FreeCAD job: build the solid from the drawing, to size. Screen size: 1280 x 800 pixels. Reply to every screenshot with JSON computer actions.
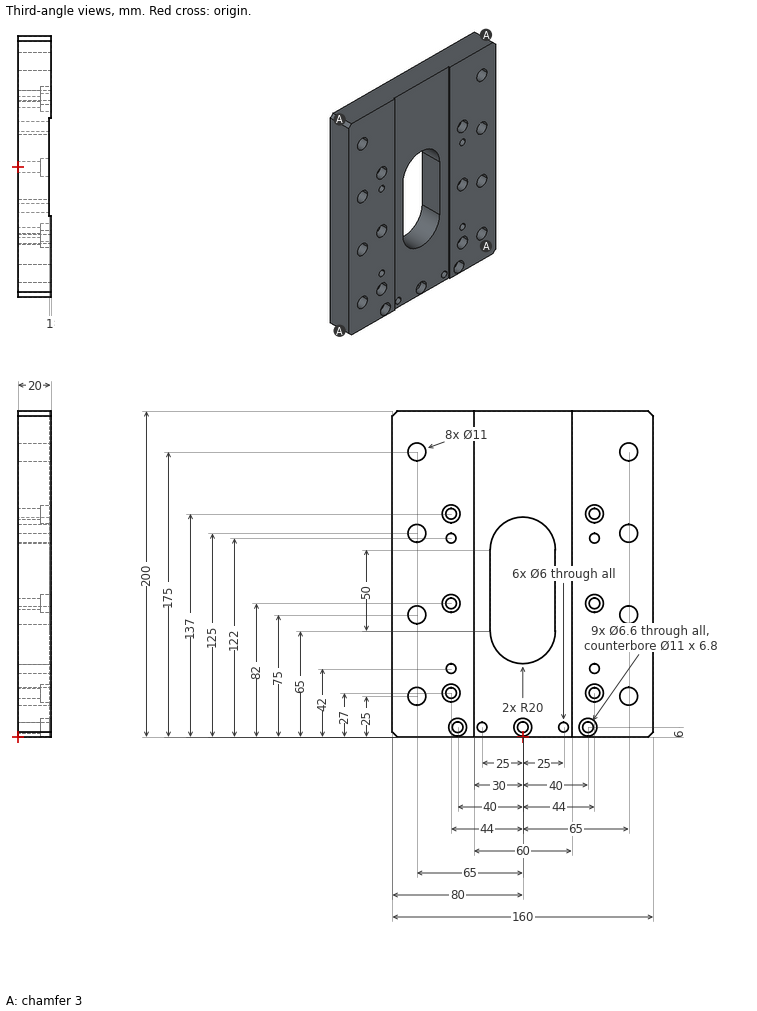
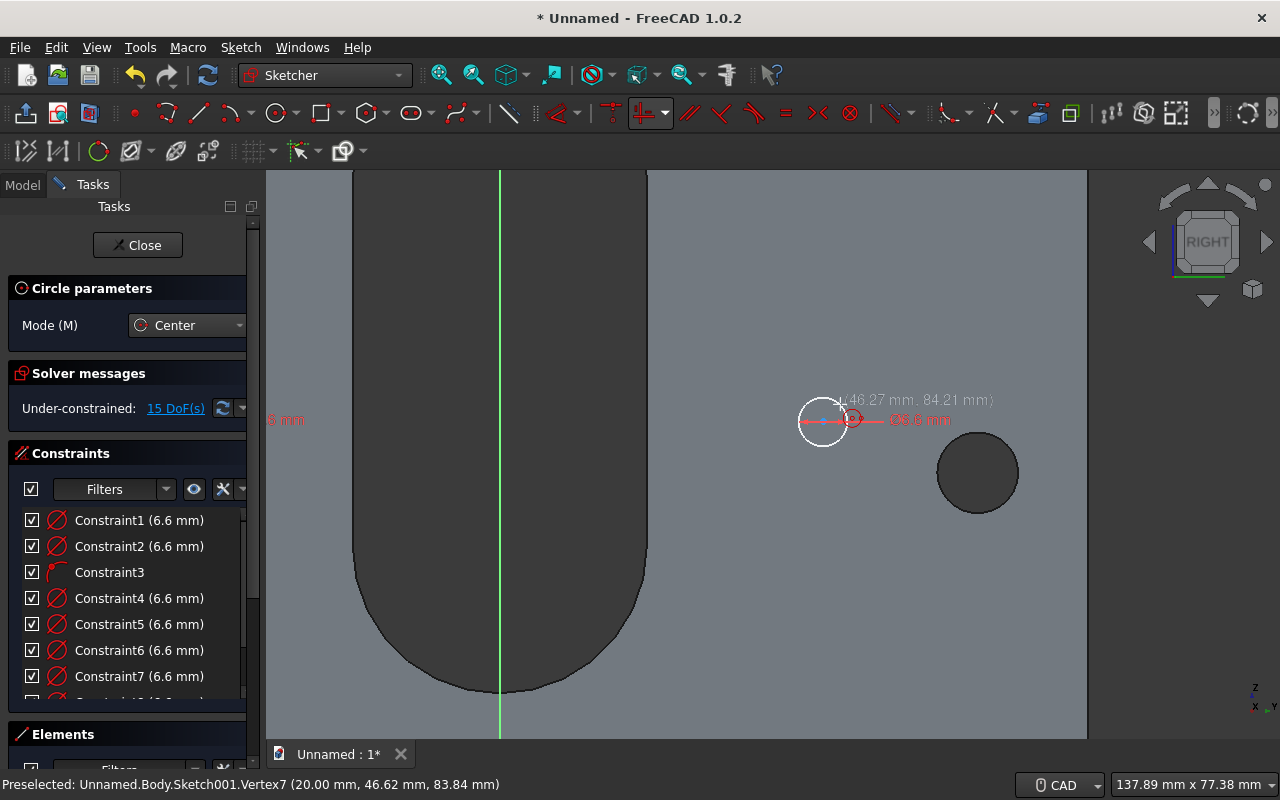
{"action": "scroll", "coordinate": [824, 423], "scroll_direction": "down", "scroll_amount": 5}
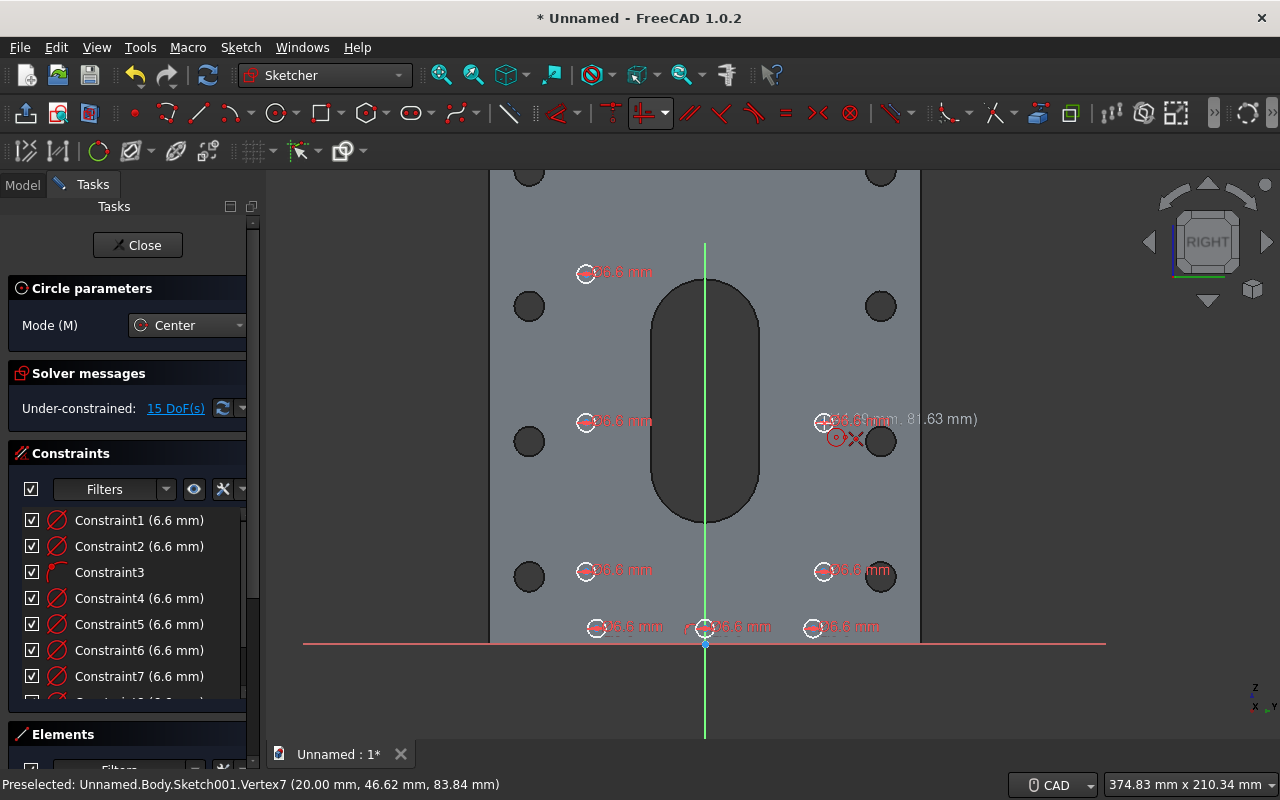
{"action": "scroll", "coordinate": [824, 274], "scroll_direction": "up", "scroll_amount": 5}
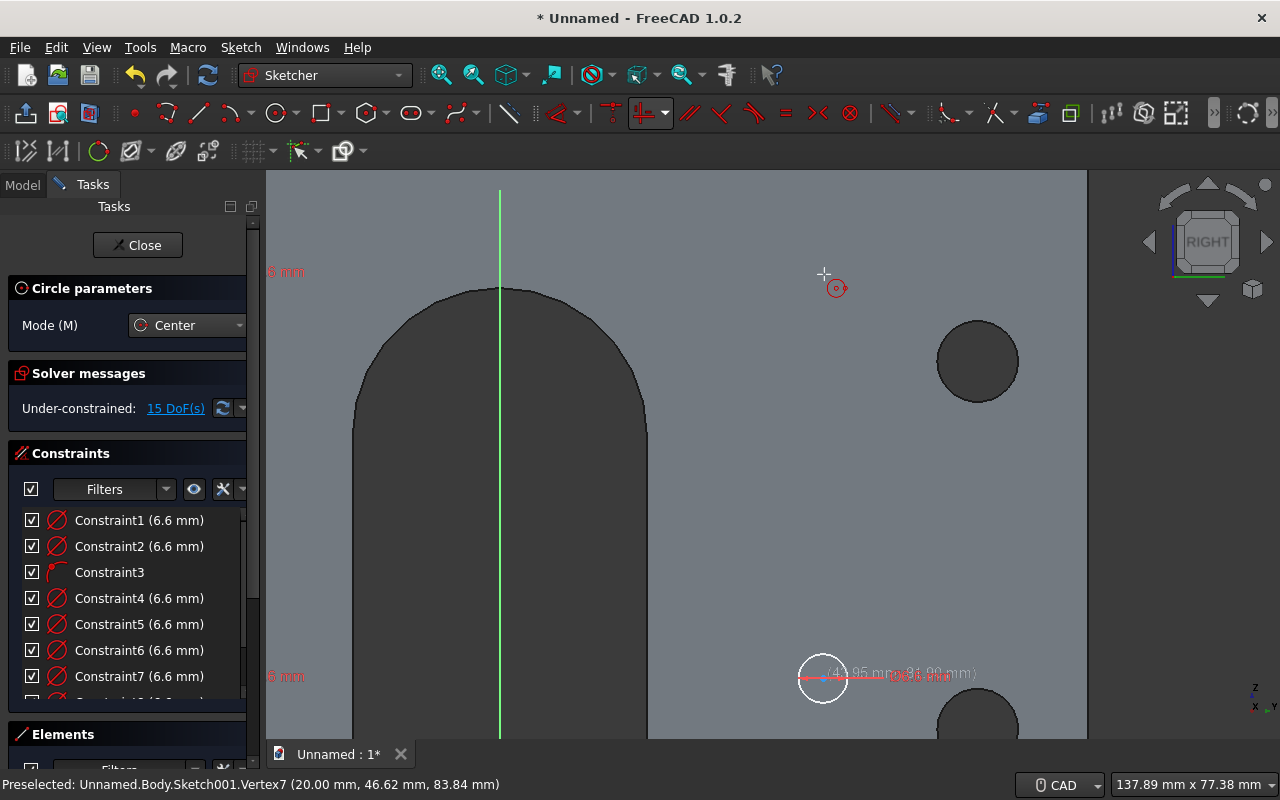
{"action": "left_click", "coordinate": [823, 273]}
{"action": "mouse_move", "coordinate": [840, 256]}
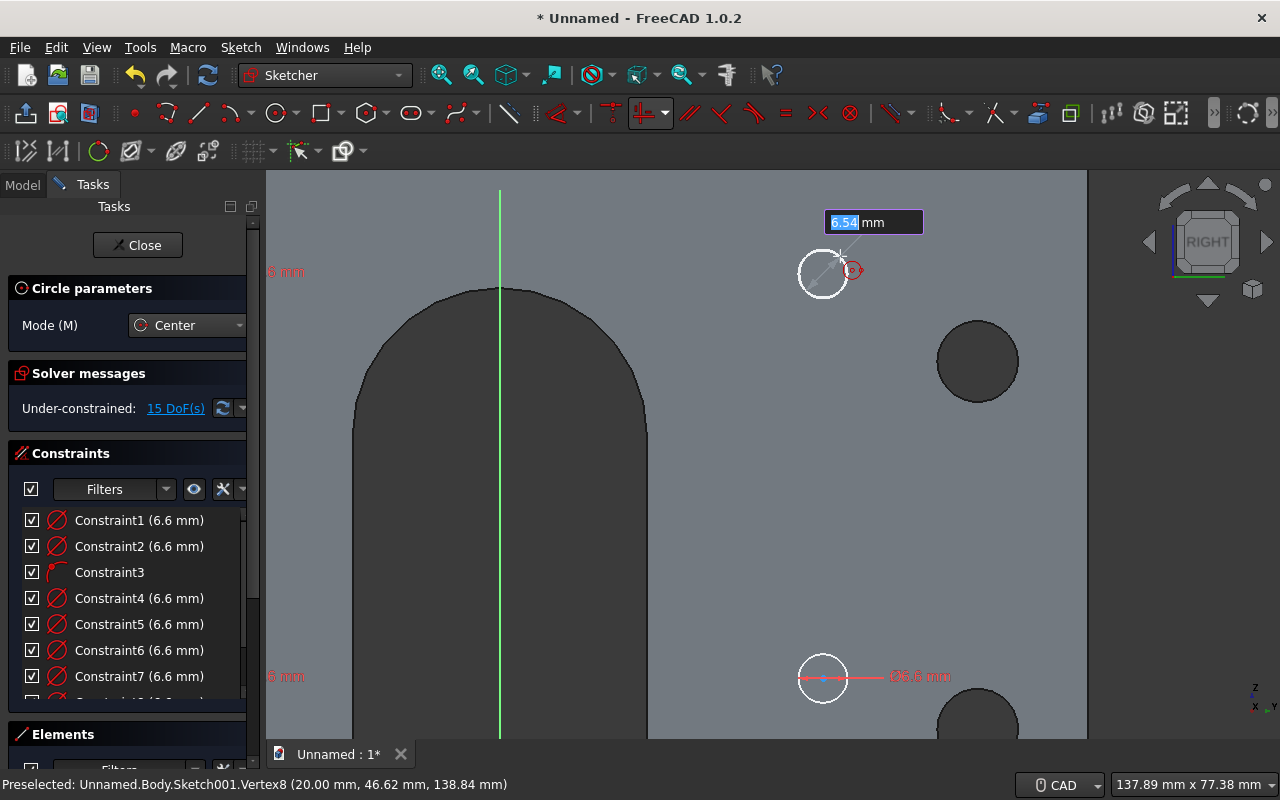
{"action": "type", "text": "6.6"}
{"action": "key", "text": "Return"}
{"action": "key", "text": "Escape"}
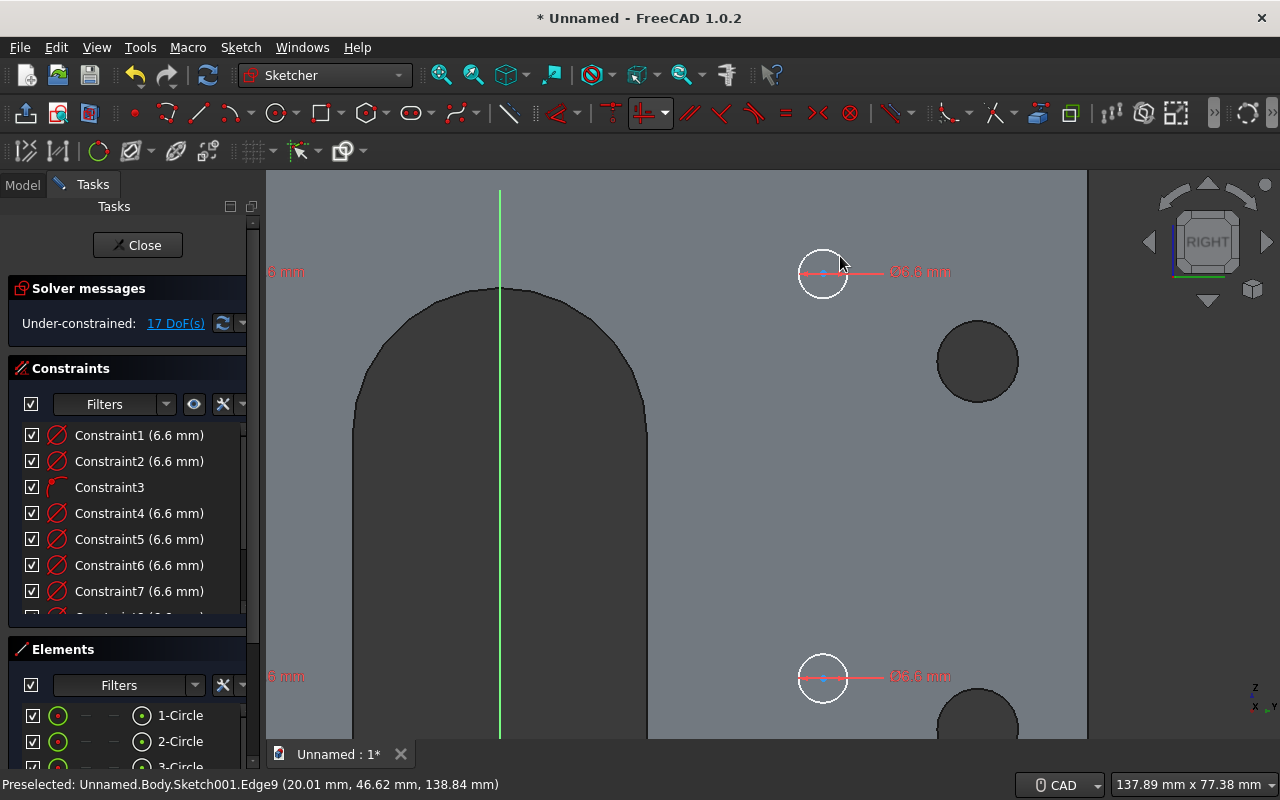
{"action": "scroll", "coordinate": [824, 274], "scroll_direction": "down", "scroll_amount": 5}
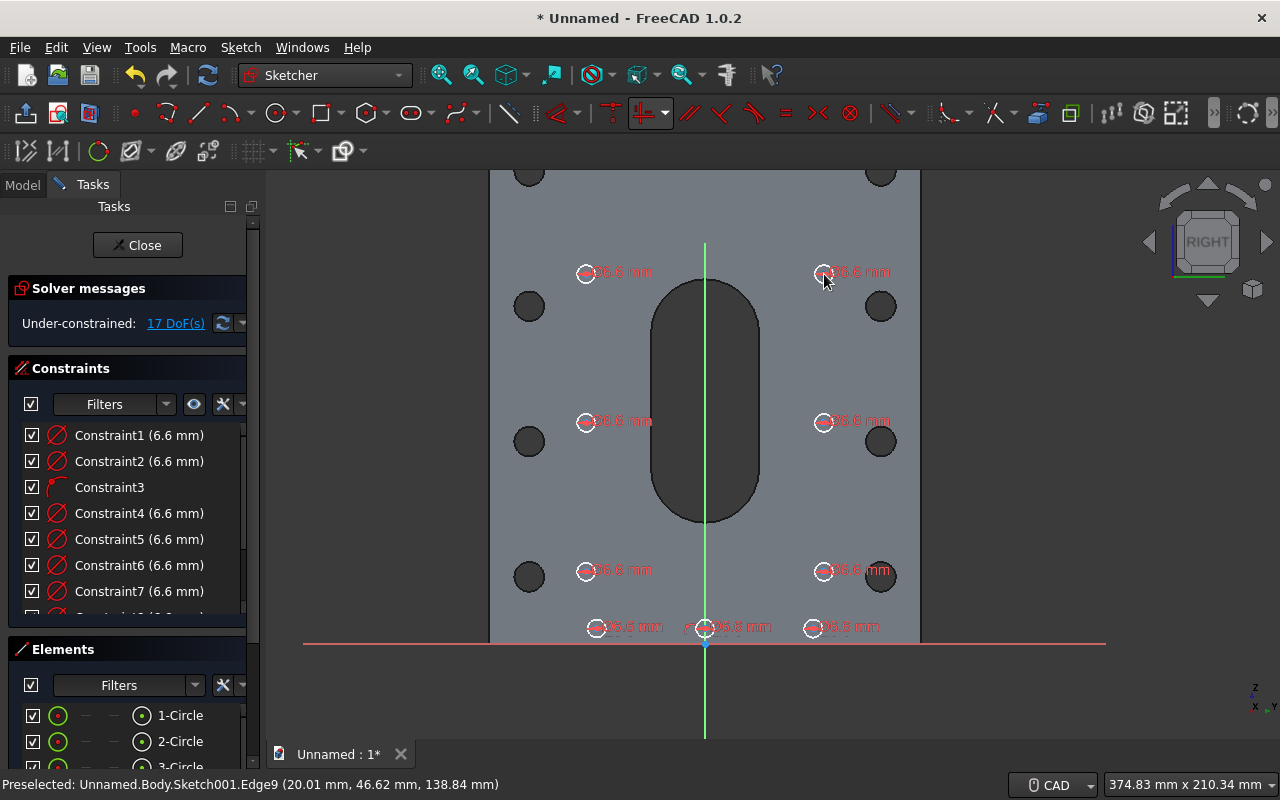
{"action": "left_click", "coordinate": [813, 629]}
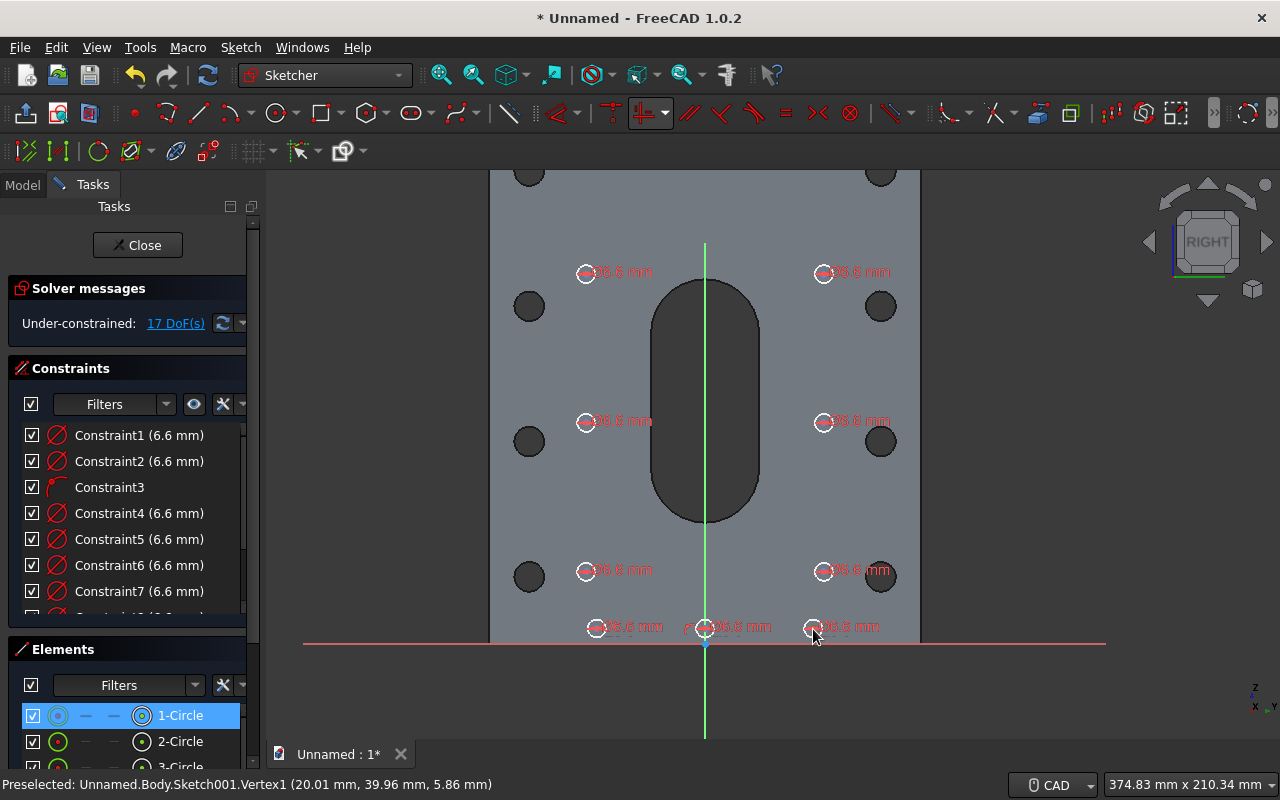
{"action": "left_click", "coordinate": [705, 629]}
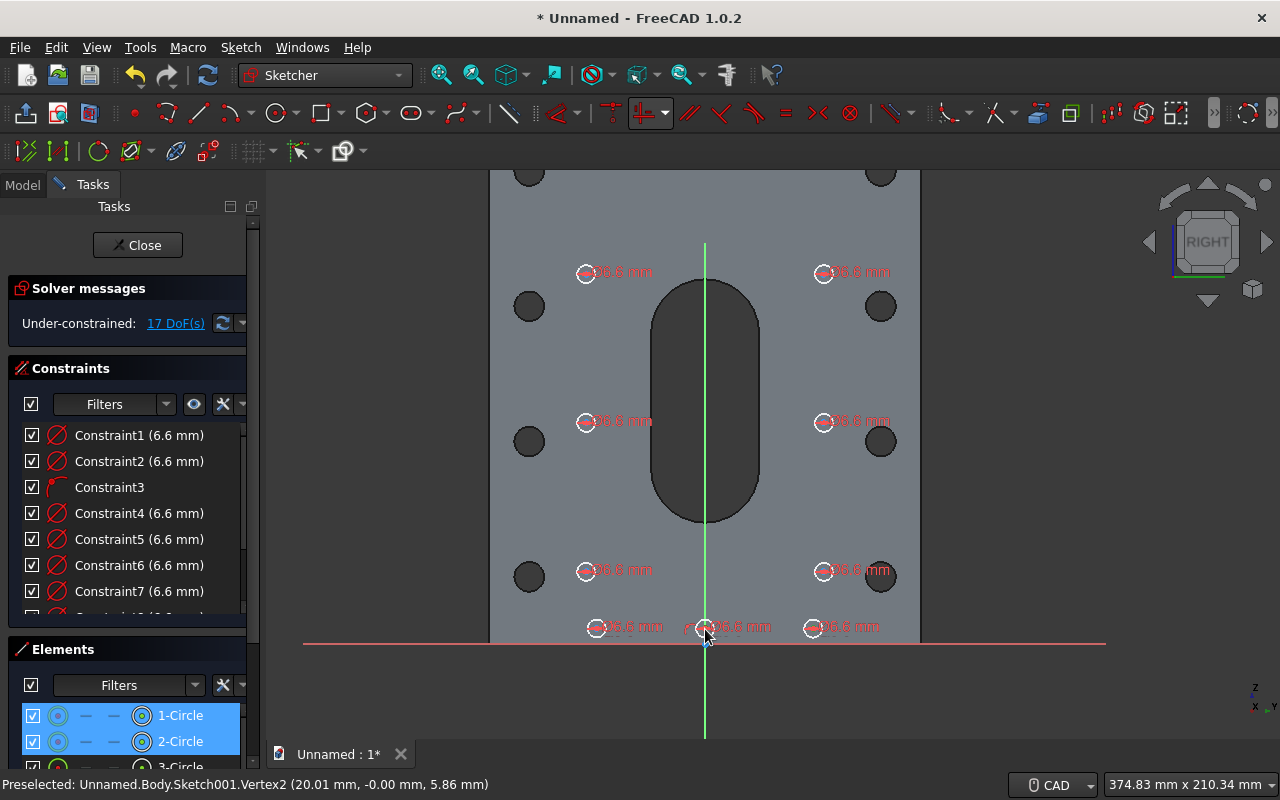
{"action": "key", "text": "h"}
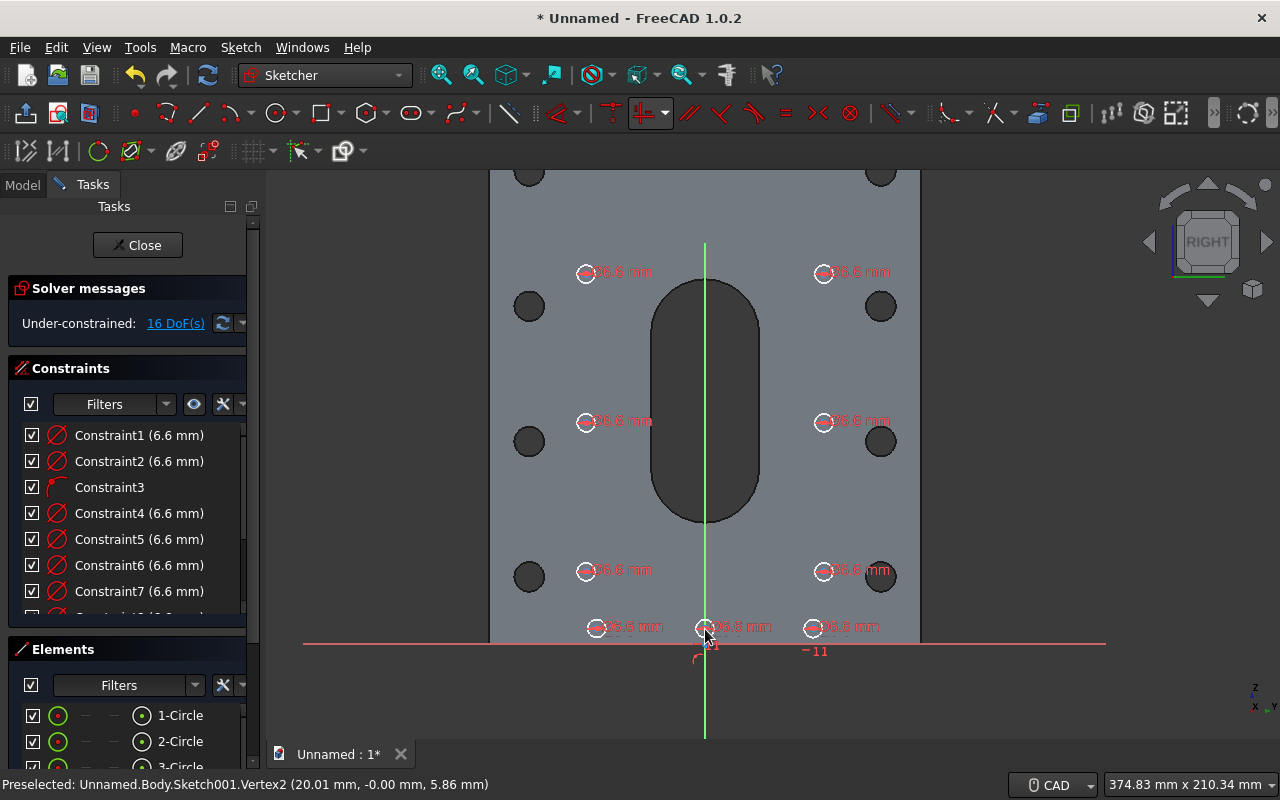
{"action": "left_click", "coordinate": [705, 629]}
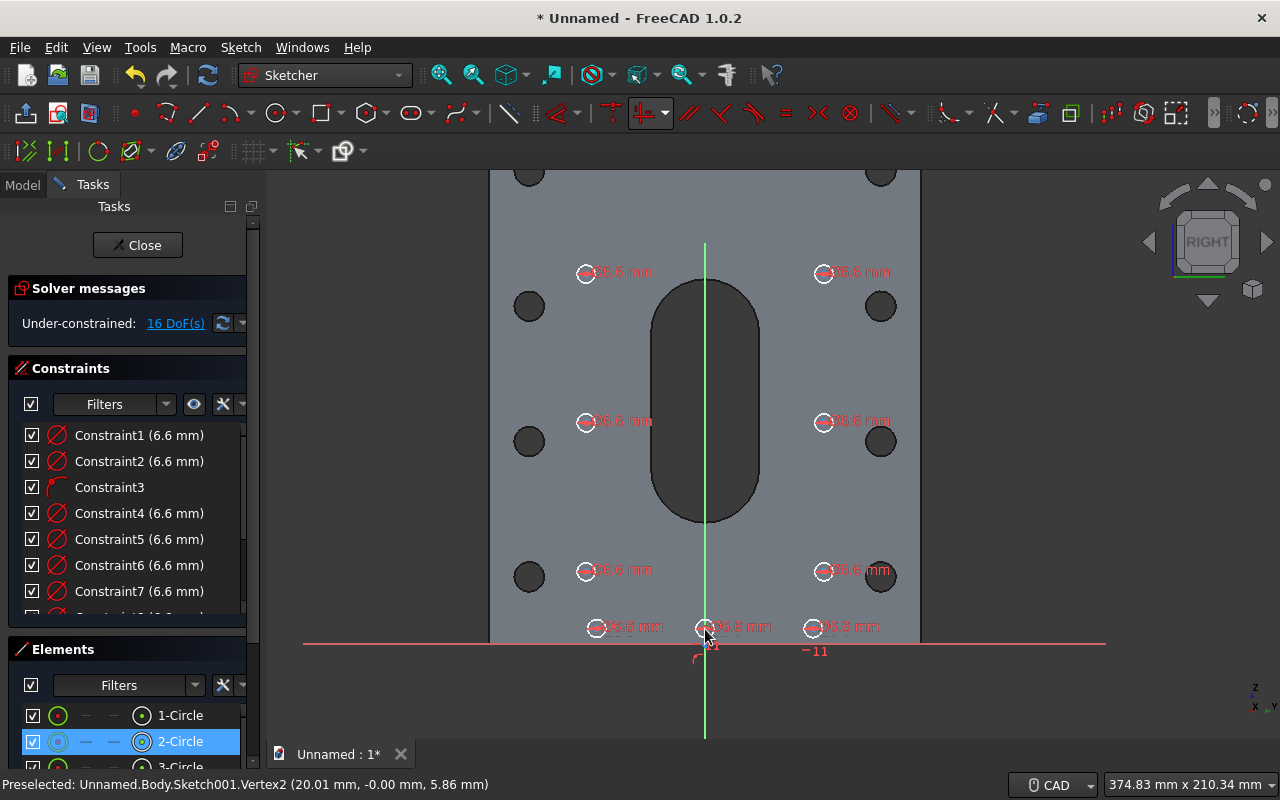
{"action": "left_click", "coordinate": [597, 629]}